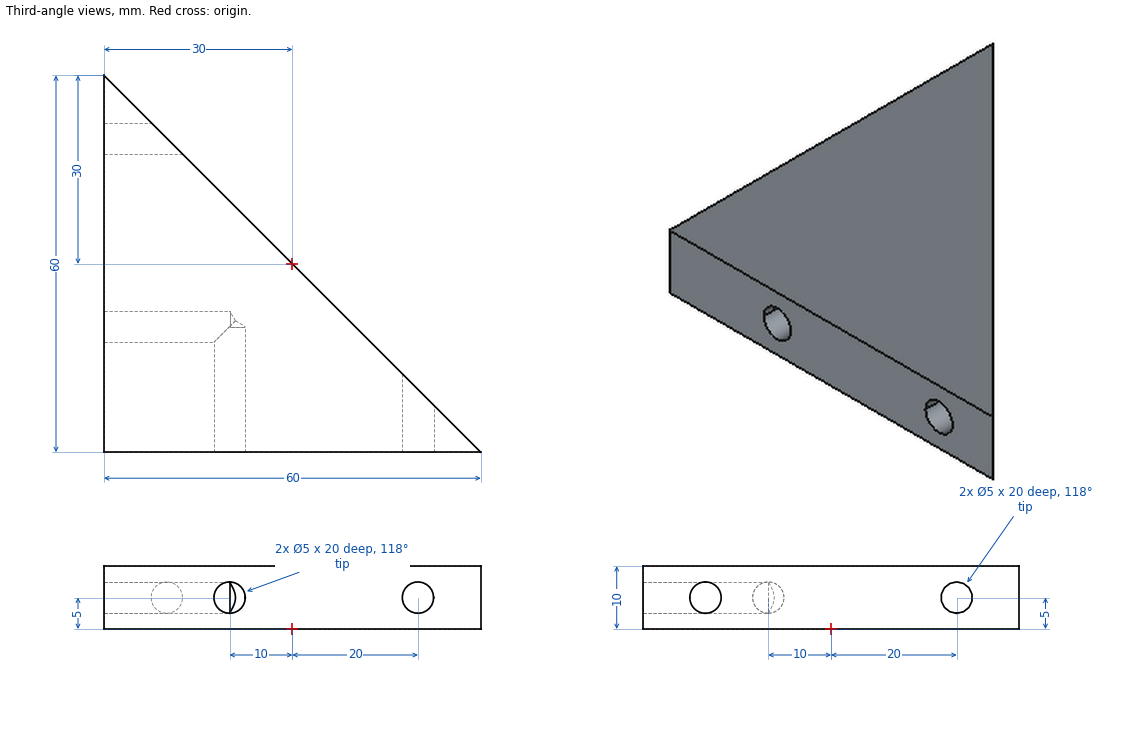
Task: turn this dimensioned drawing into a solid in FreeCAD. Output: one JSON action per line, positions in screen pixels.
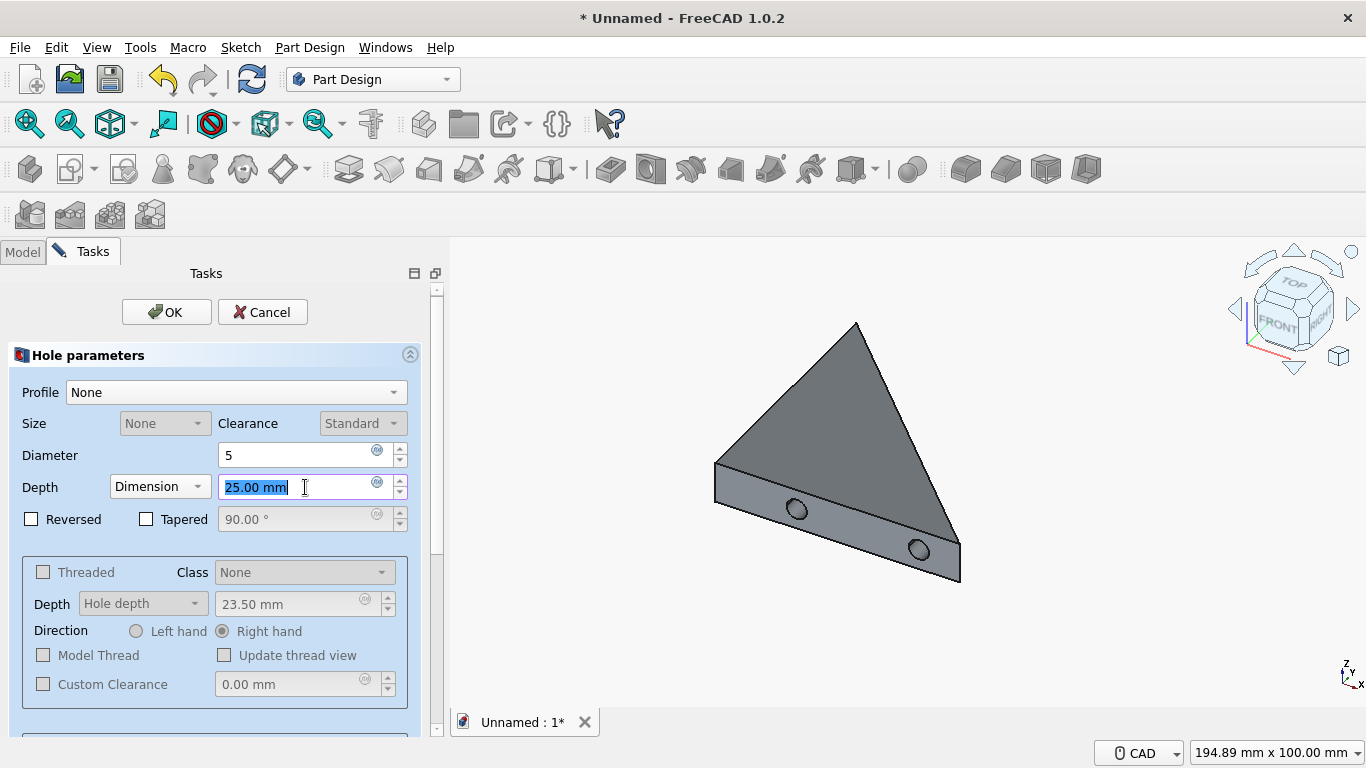
{"action": "type", "text": "20"}
{"action": "key", "text": "Tab"}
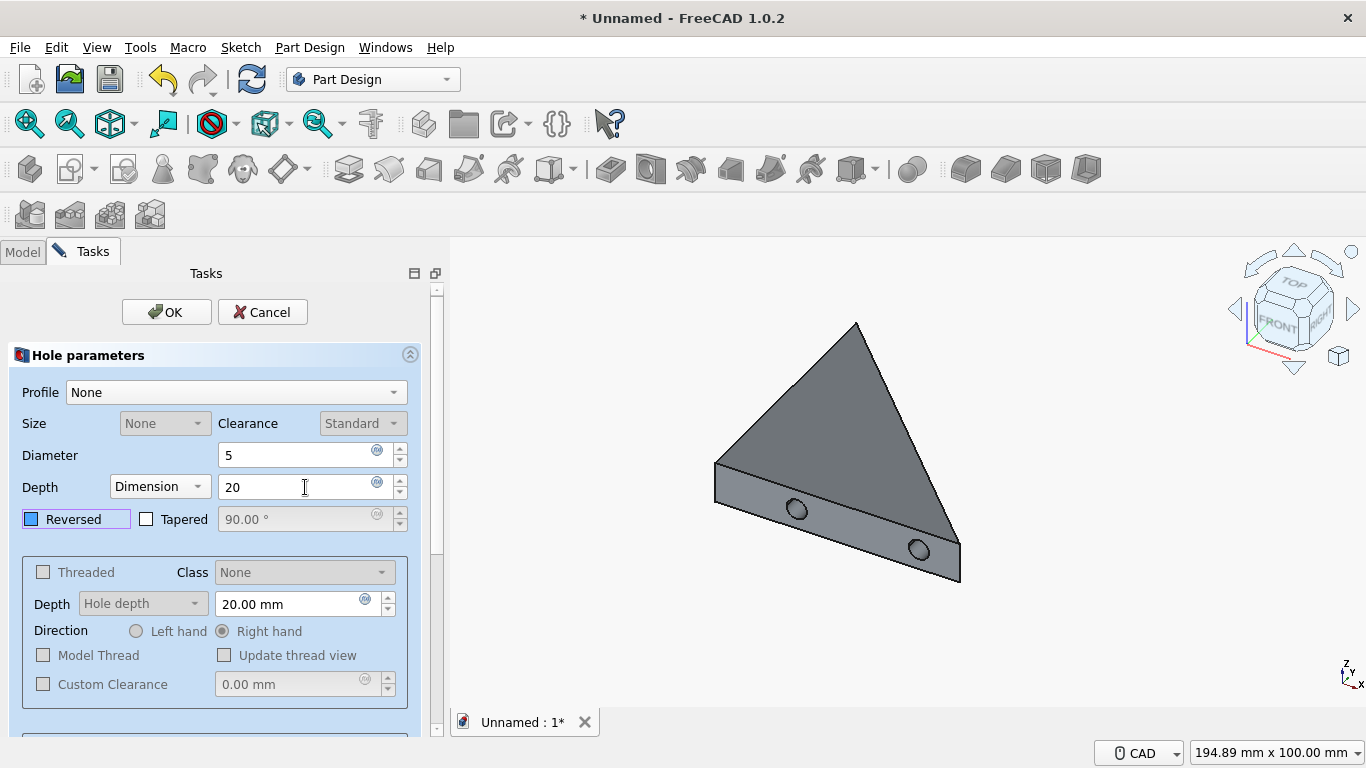
{"action": "left_click", "coordinate": [167, 312]}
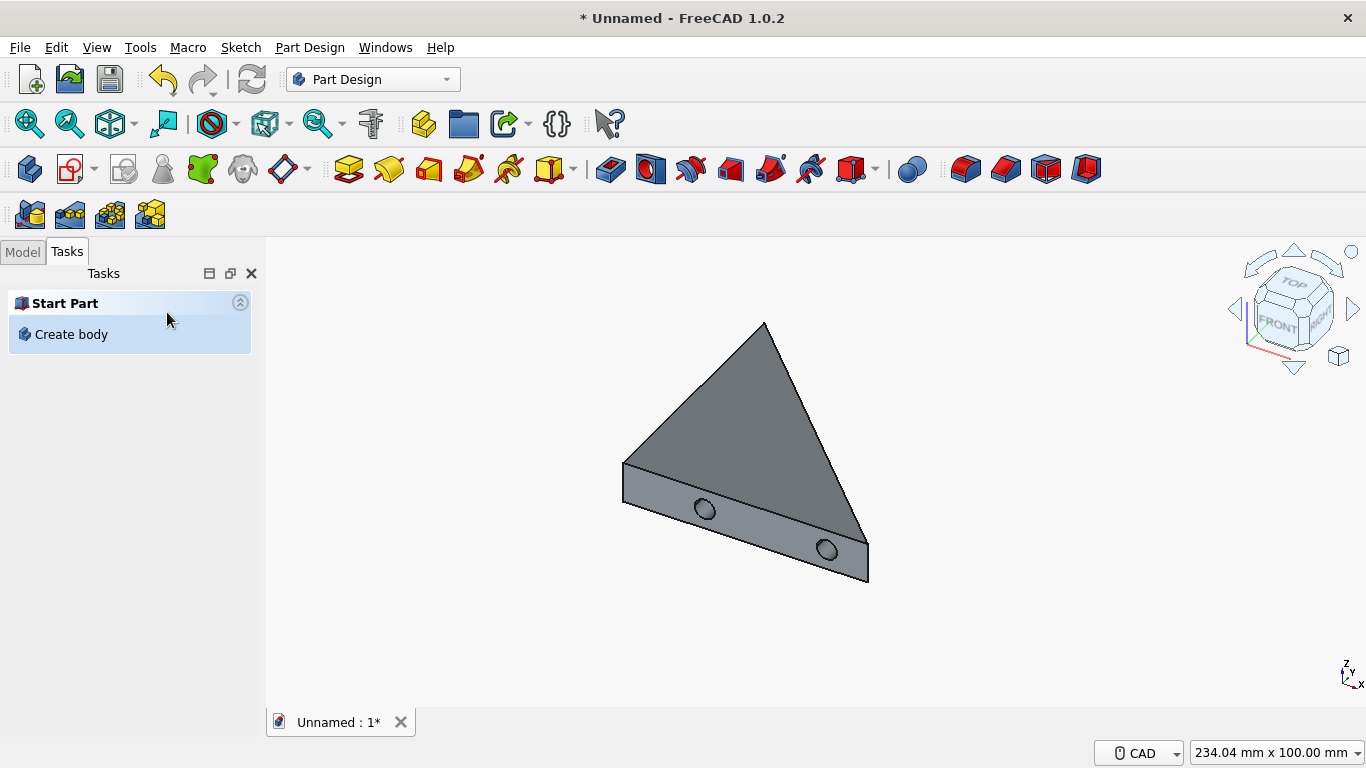
{"action": "key", "text": "6"}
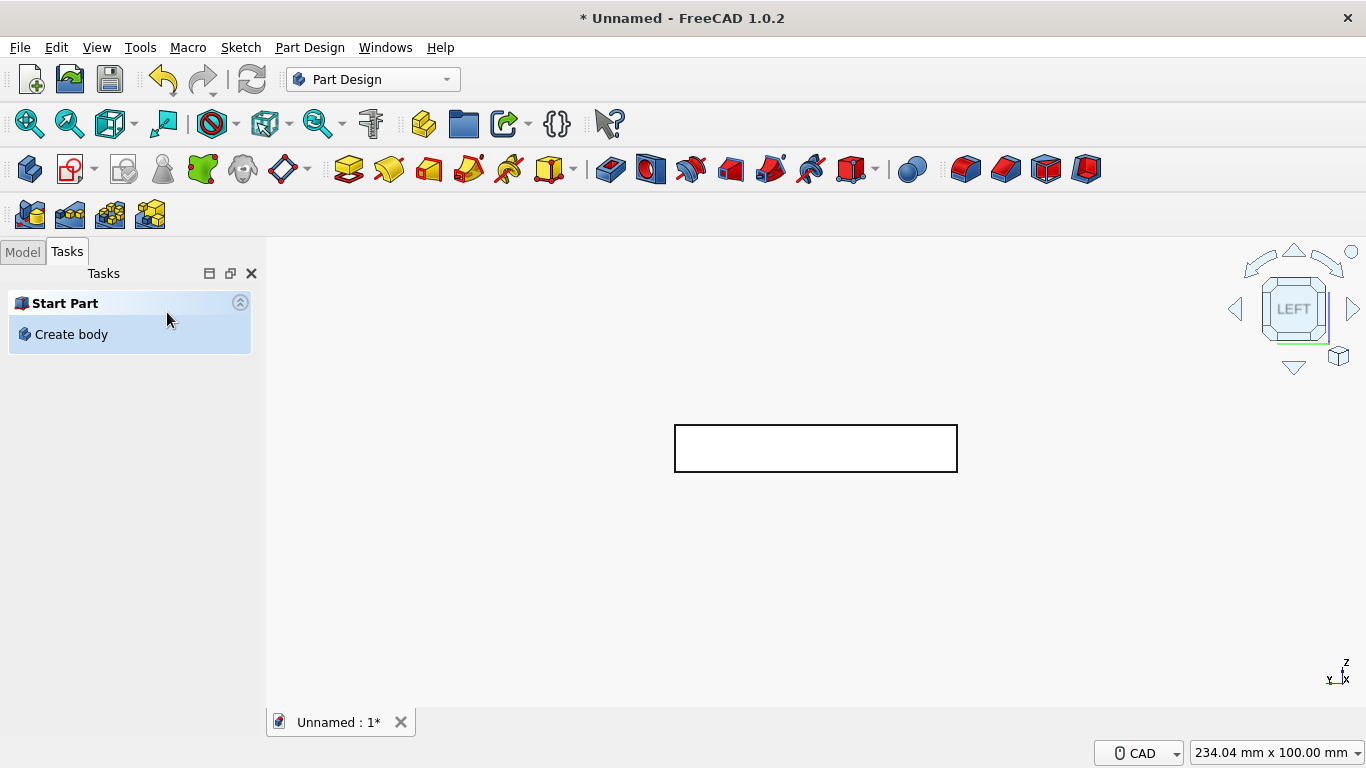
{"action": "left_click", "coordinate": [30, 124]}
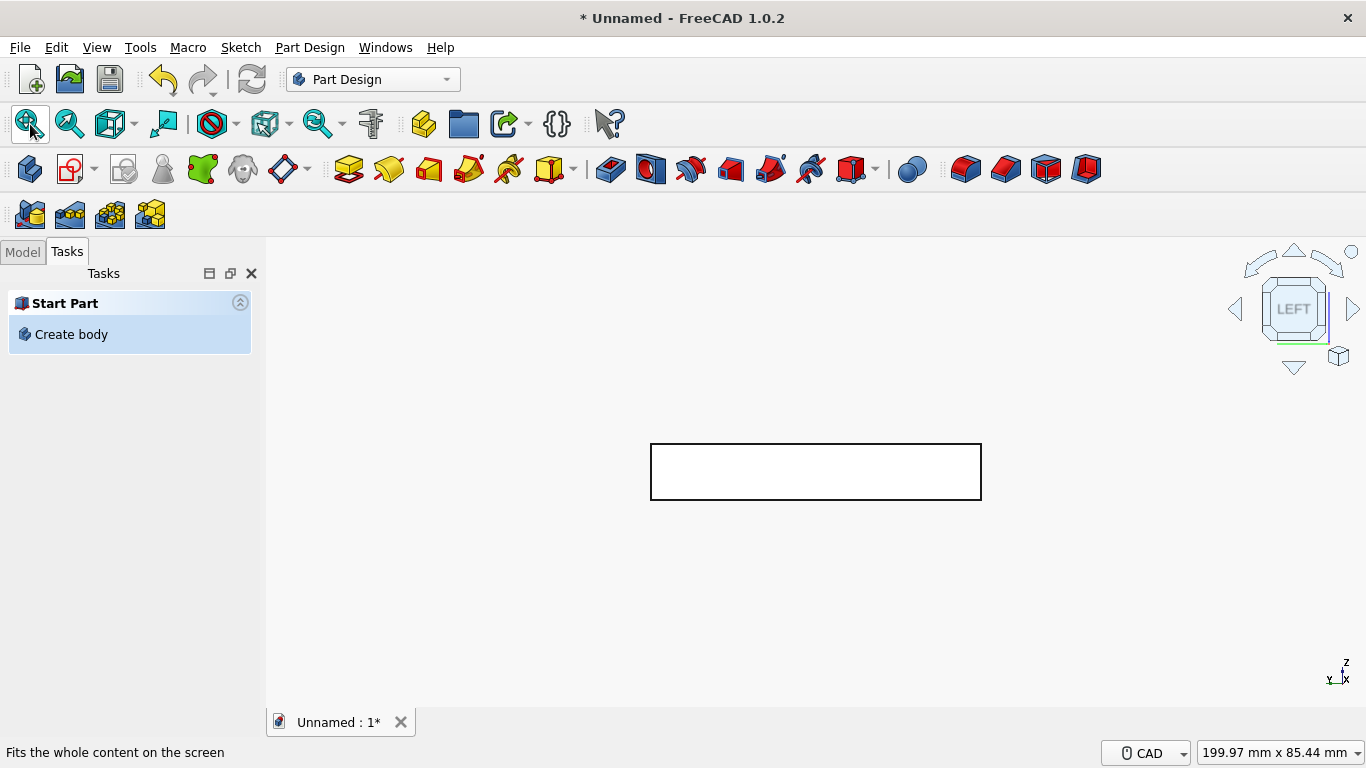
{"action": "left_click", "coordinate": [722, 471]}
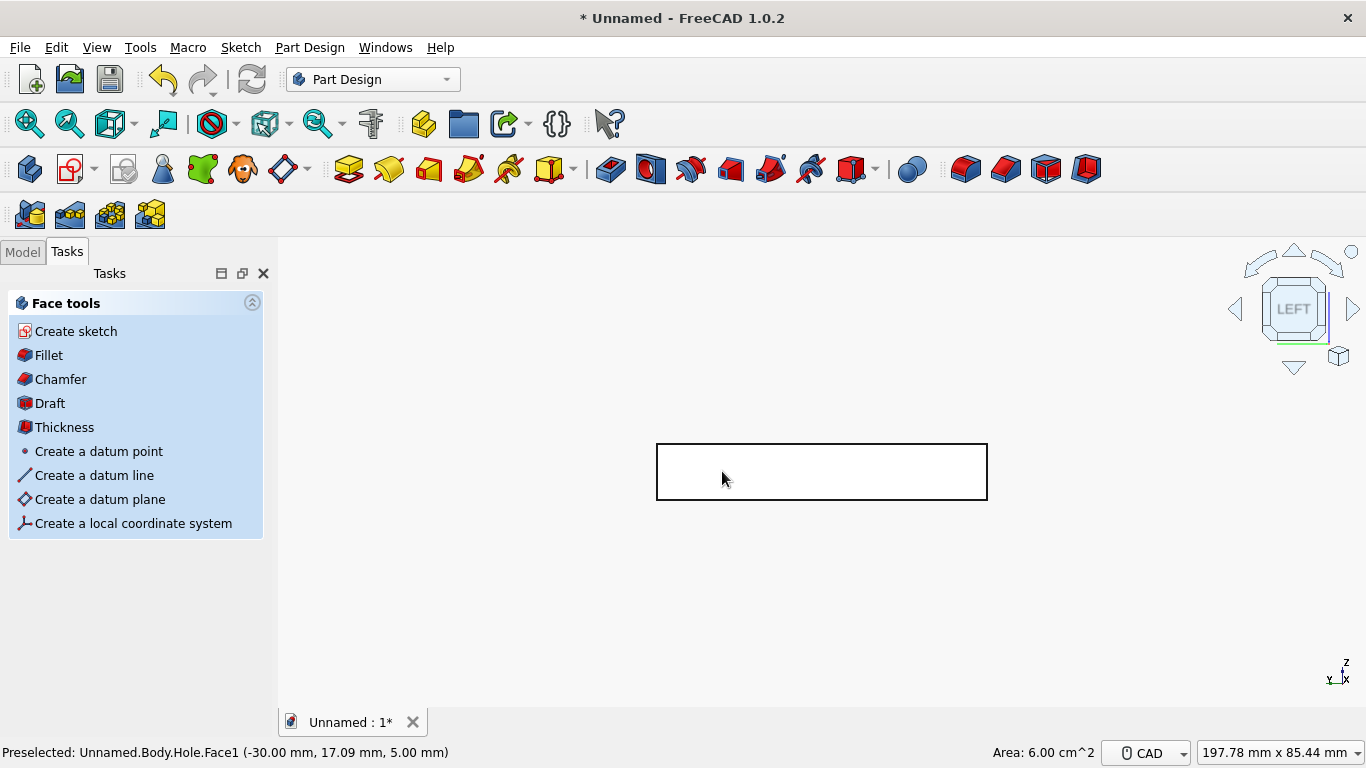
{"action": "left_click", "coordinate": [70, 170]}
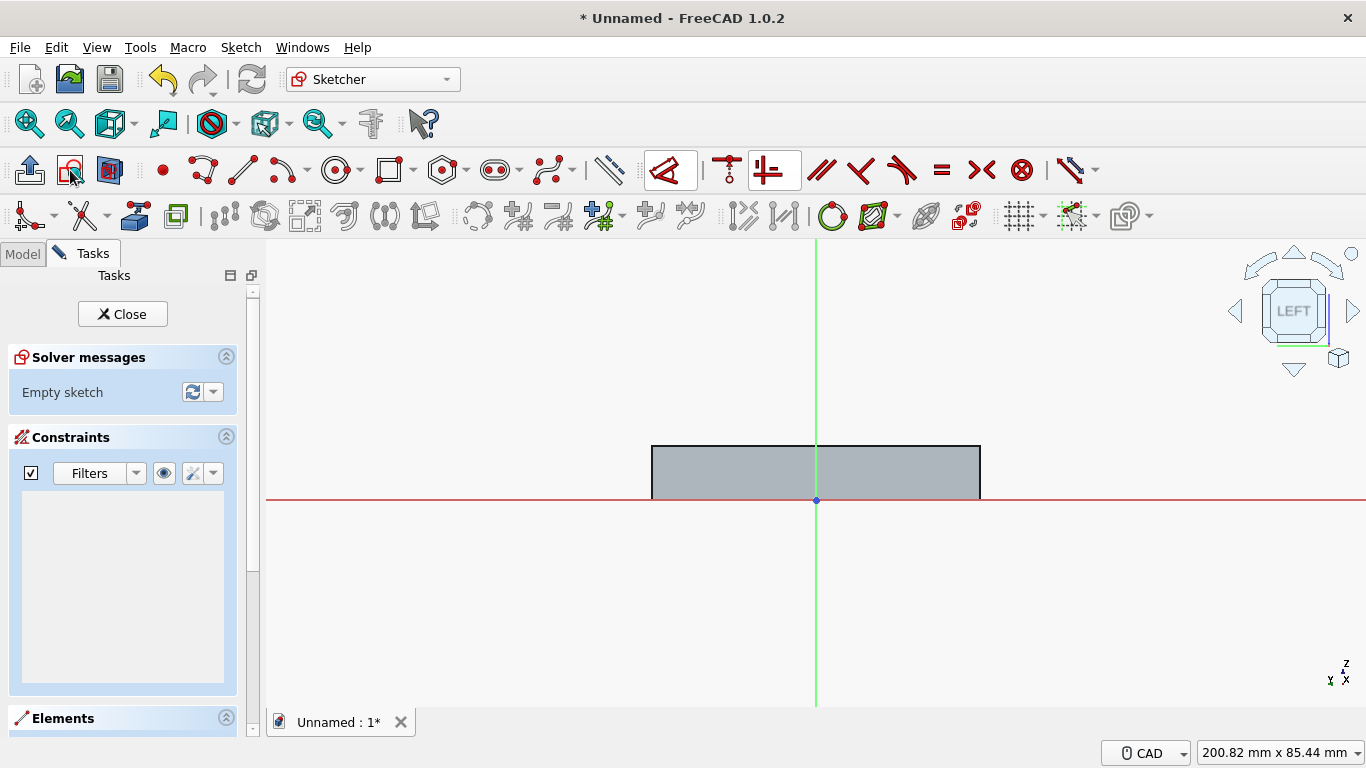
{"action": "scroll", "coordinate": [806, 483], "scroll_direction": "up", "scroll_amount": 6}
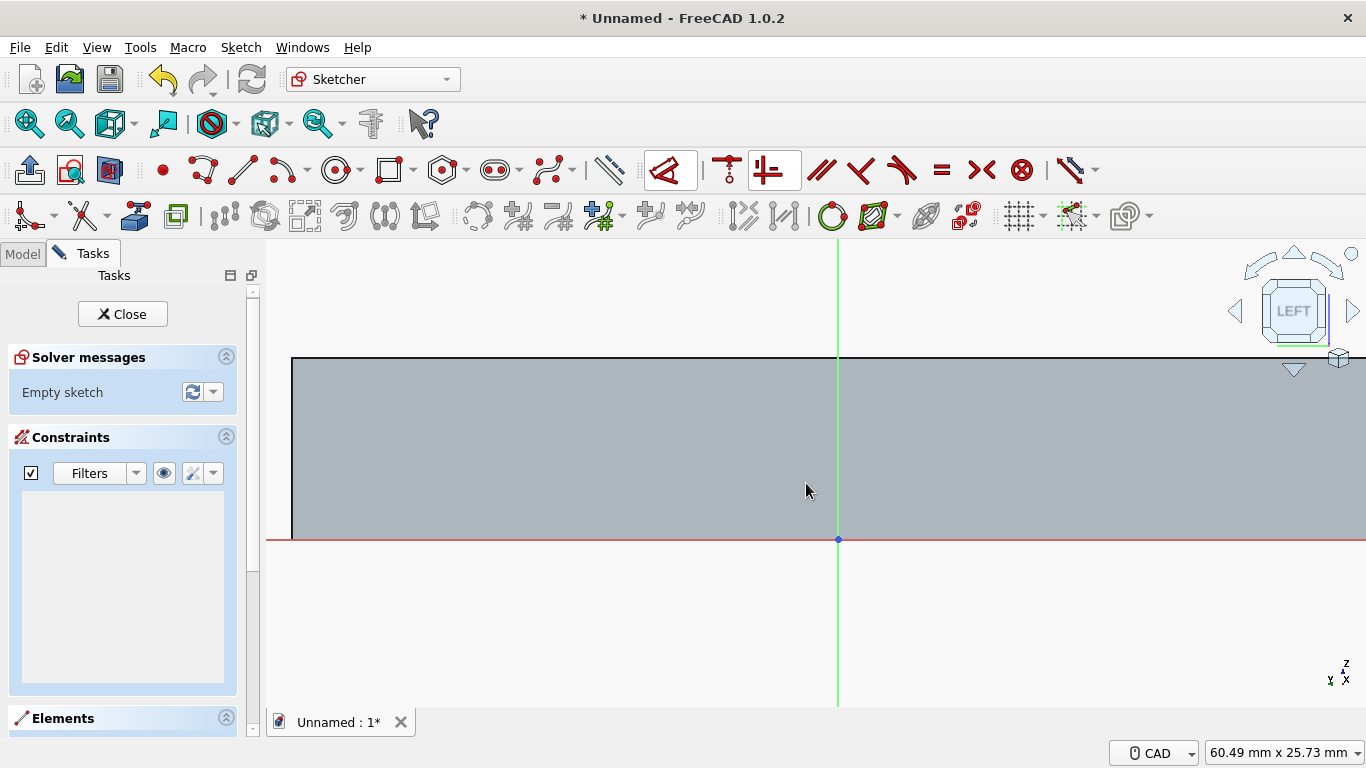
{"action": "left_click", "coordinate": [336, 170]}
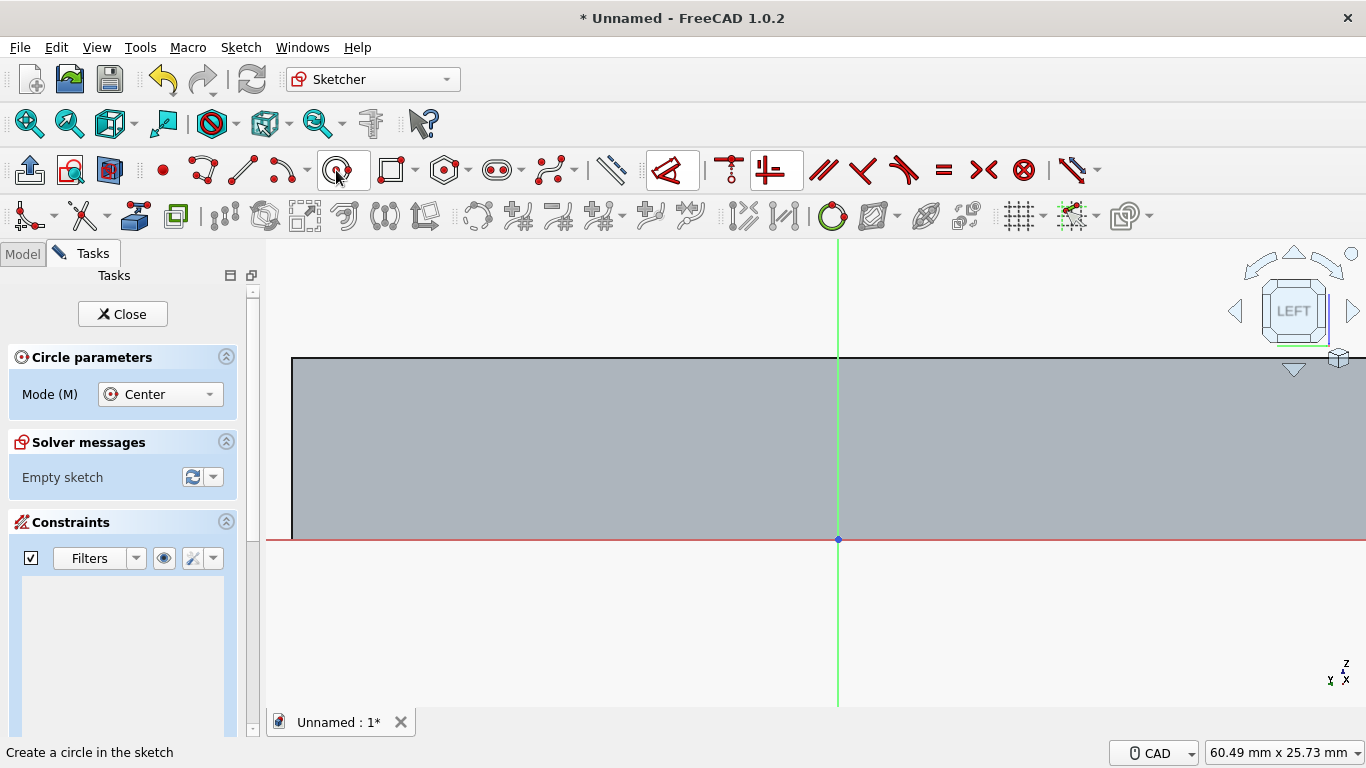
{"action": "left_click", "coordinate": [474, 449]}
{"action": "mouse_move", "coordinate": [506, 416]}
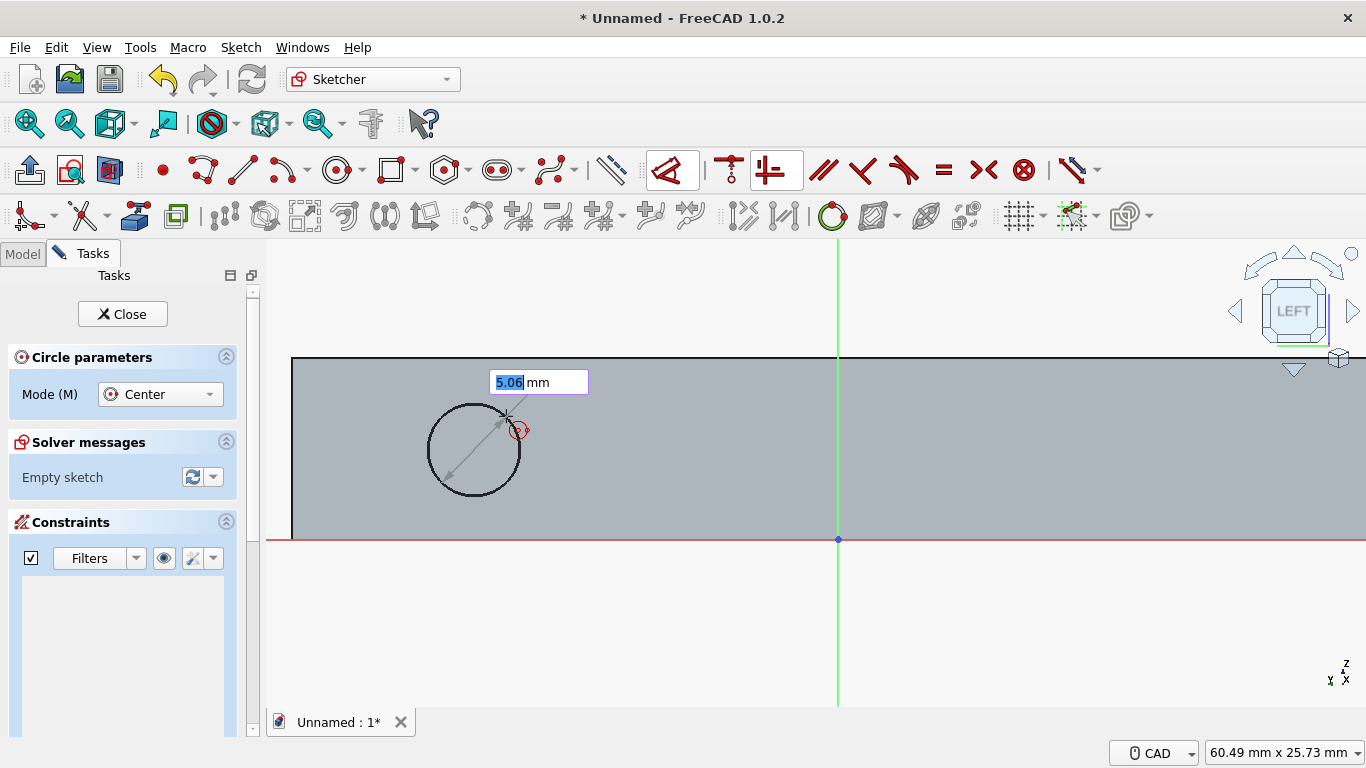
{"action": "type", "text": "5"}
{"action": "key", "text": "Return"}